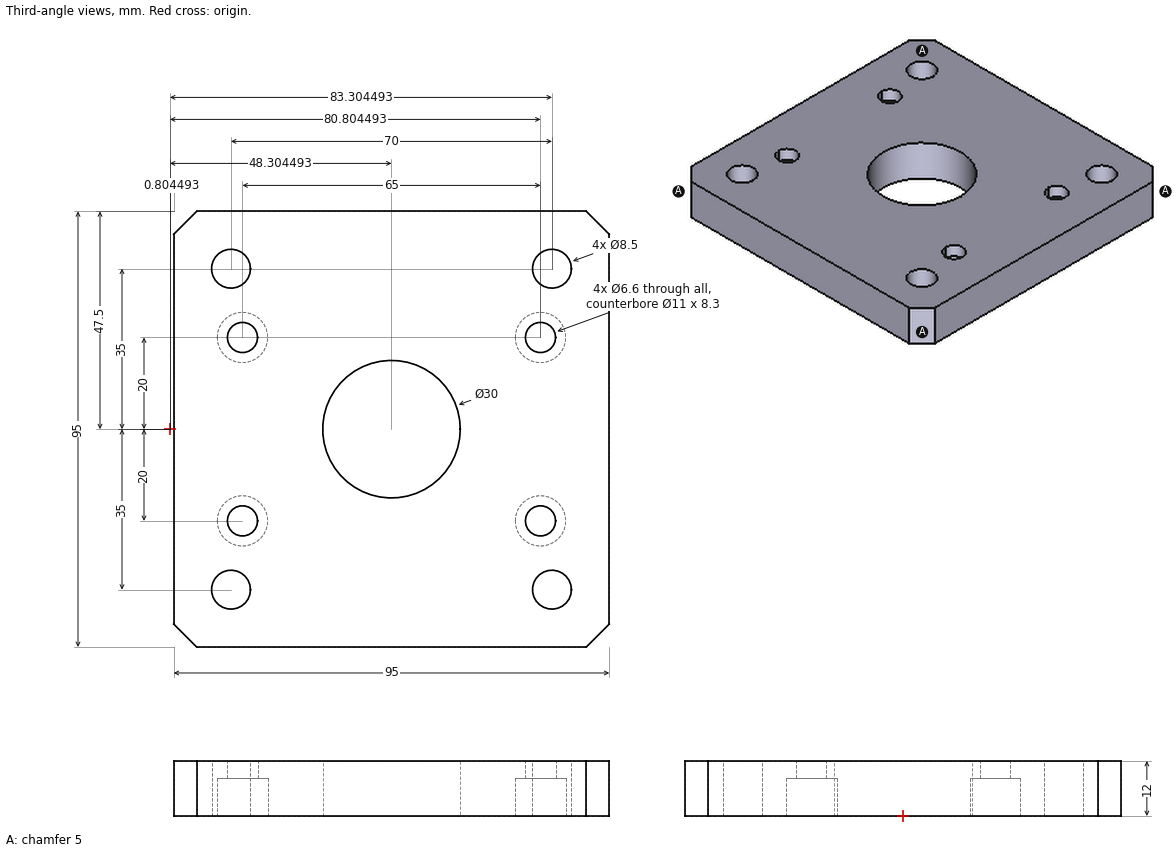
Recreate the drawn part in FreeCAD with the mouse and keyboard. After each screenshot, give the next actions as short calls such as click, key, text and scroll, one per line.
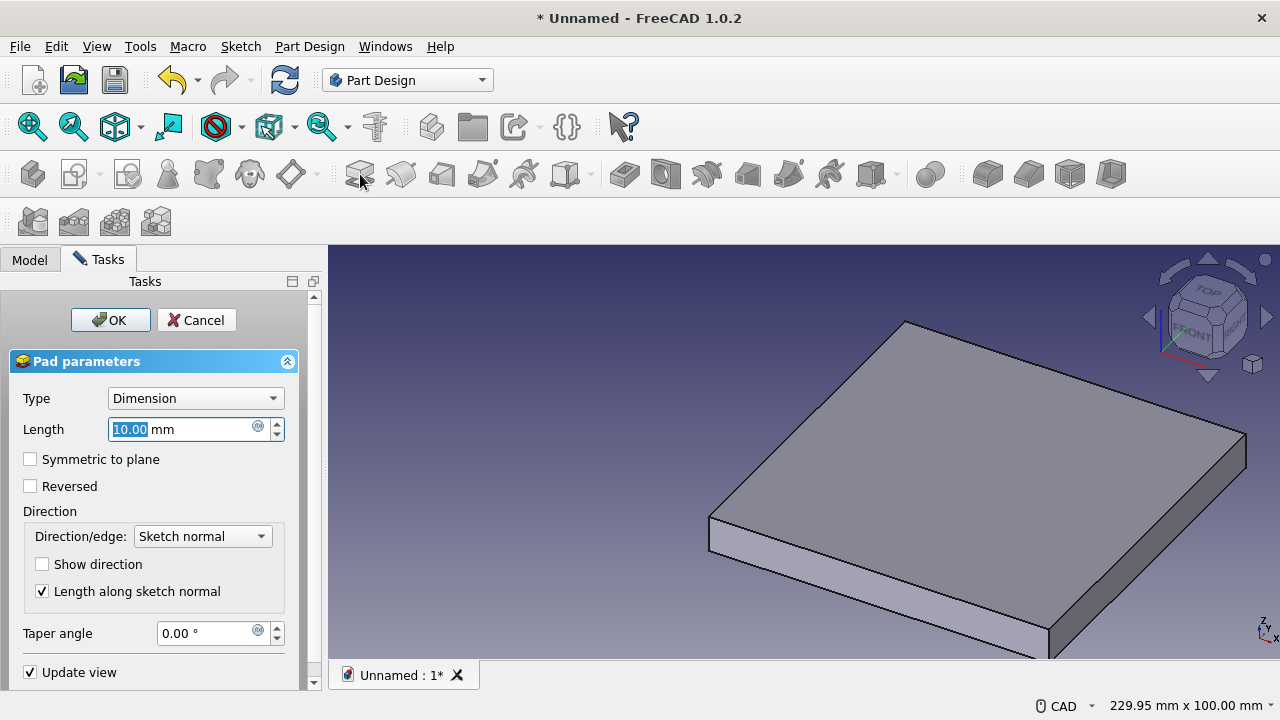
text(12)
key(Tab)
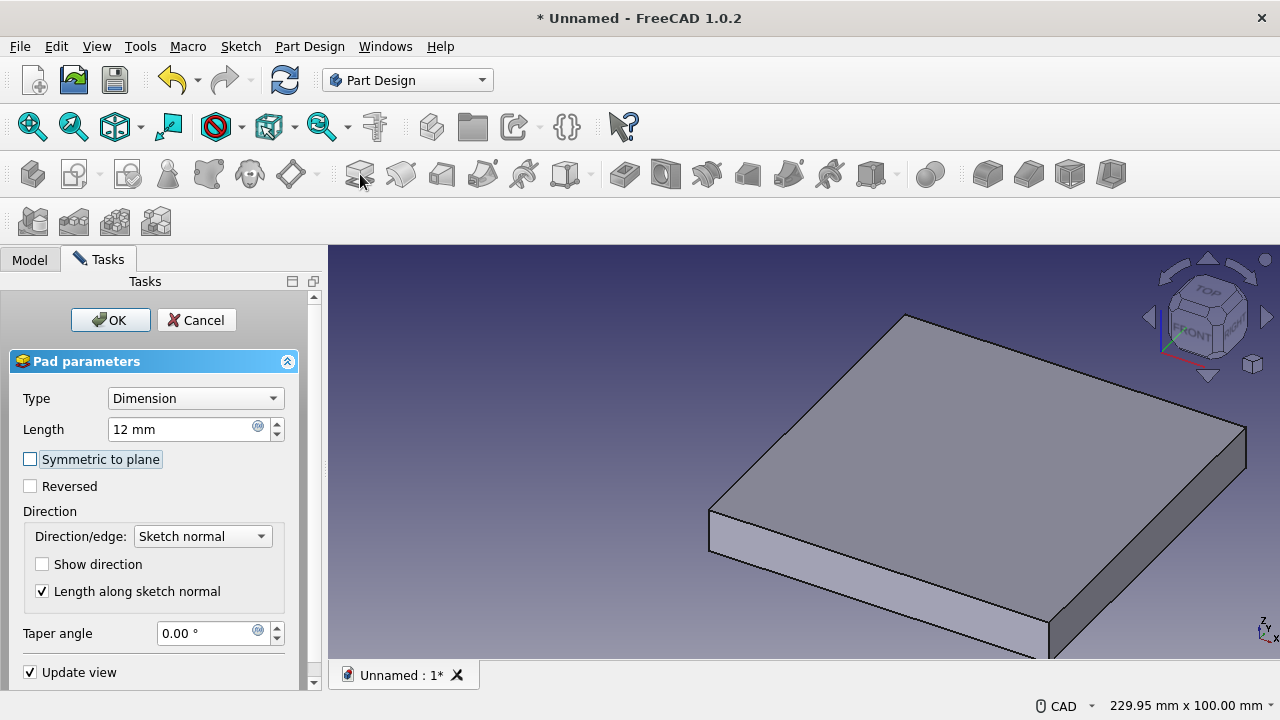
click(111, 320)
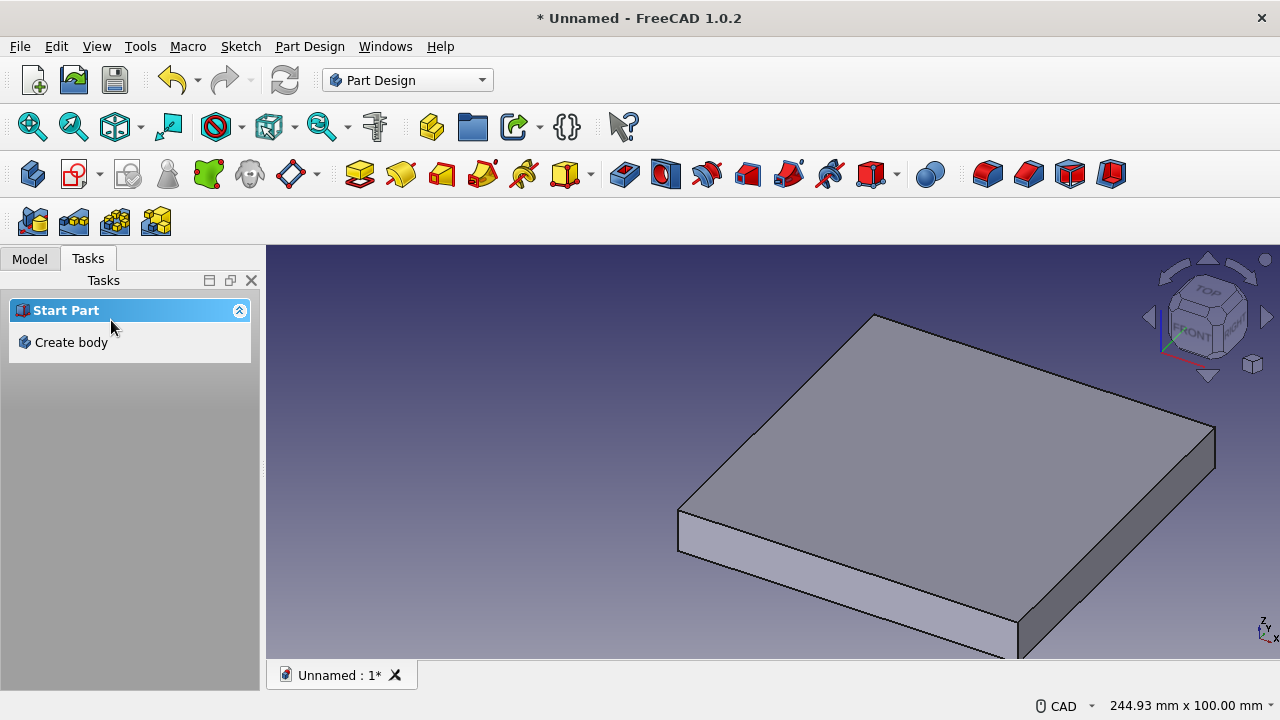
key(v)
key(f)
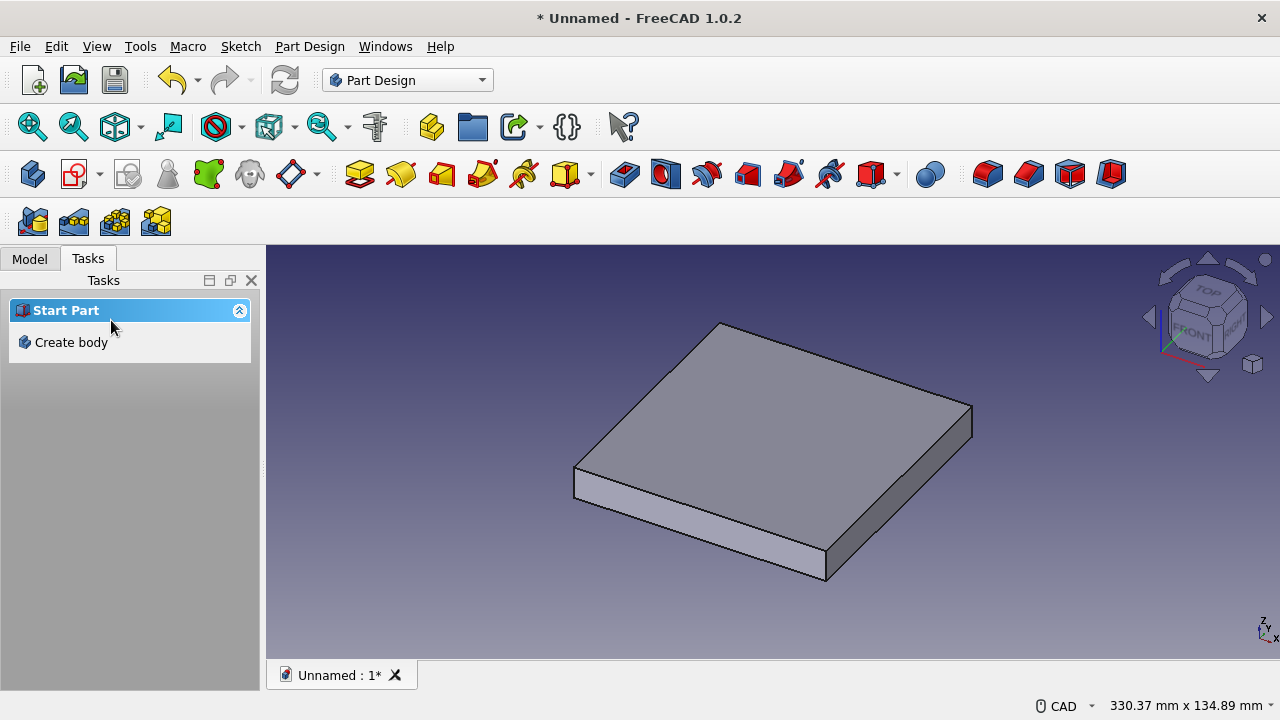
click(773, 436)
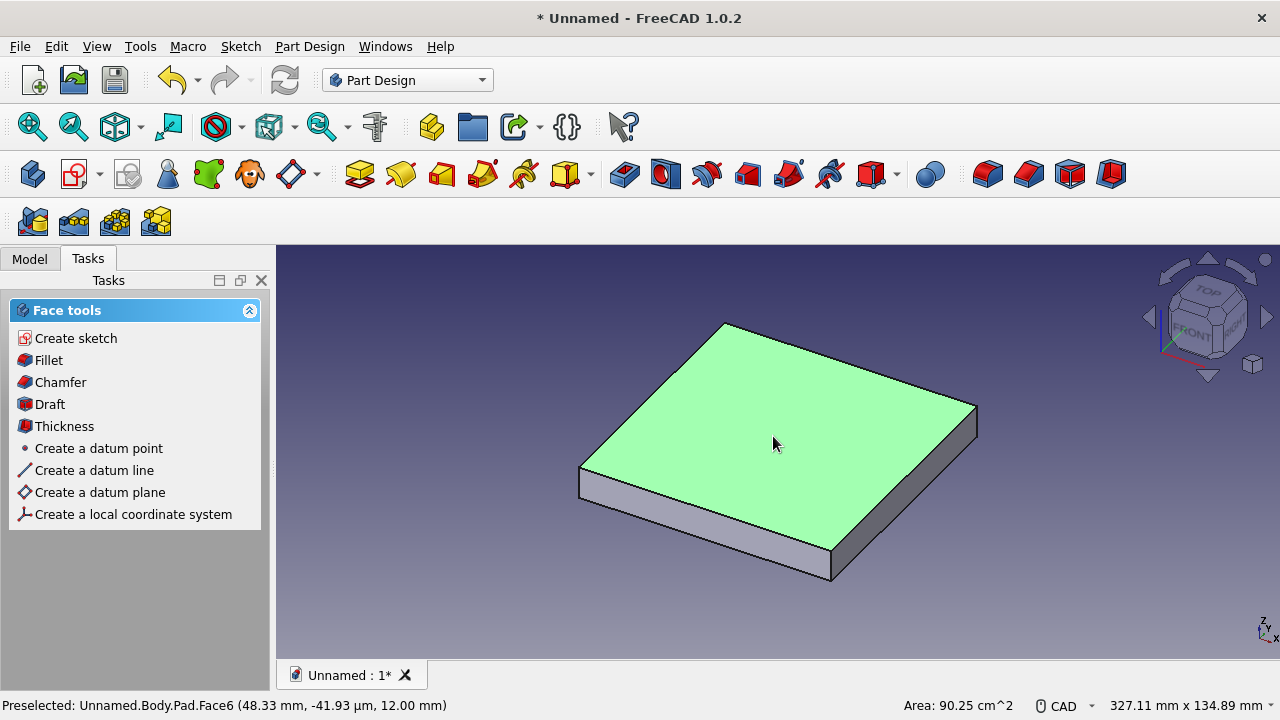
click(74, 174)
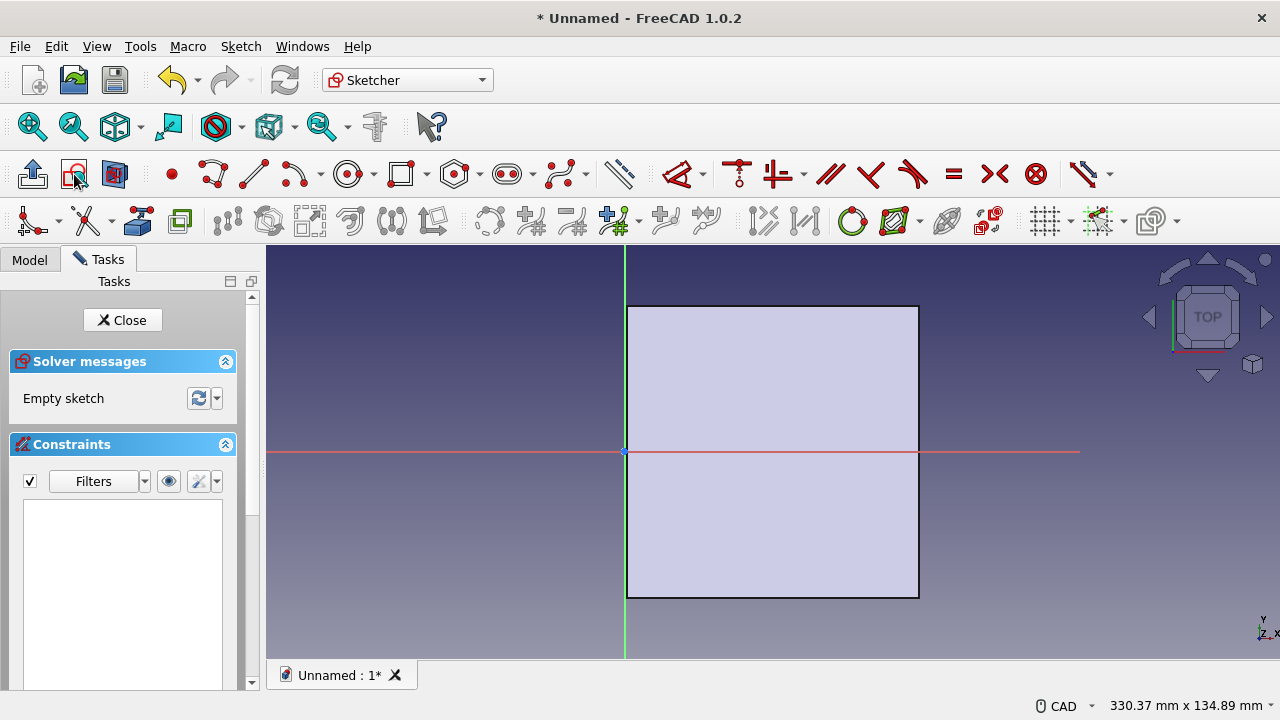
scroll(732, 452, up, 5)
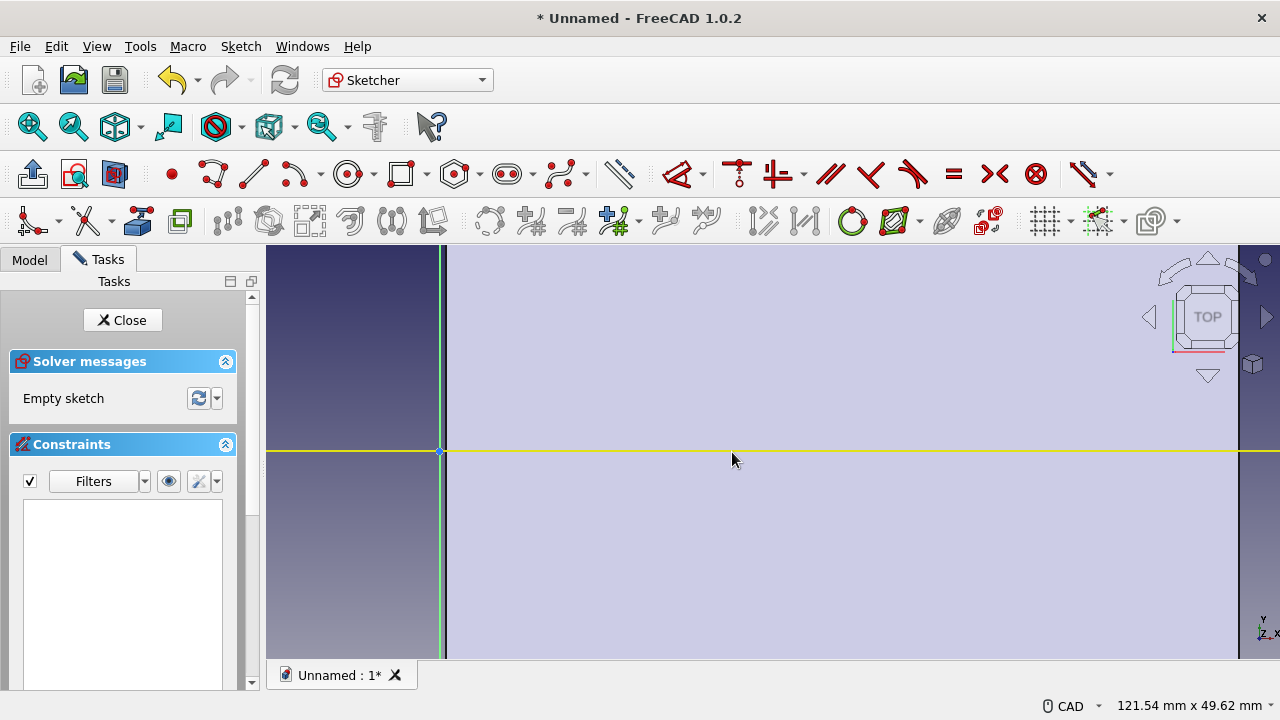
click(348, 174)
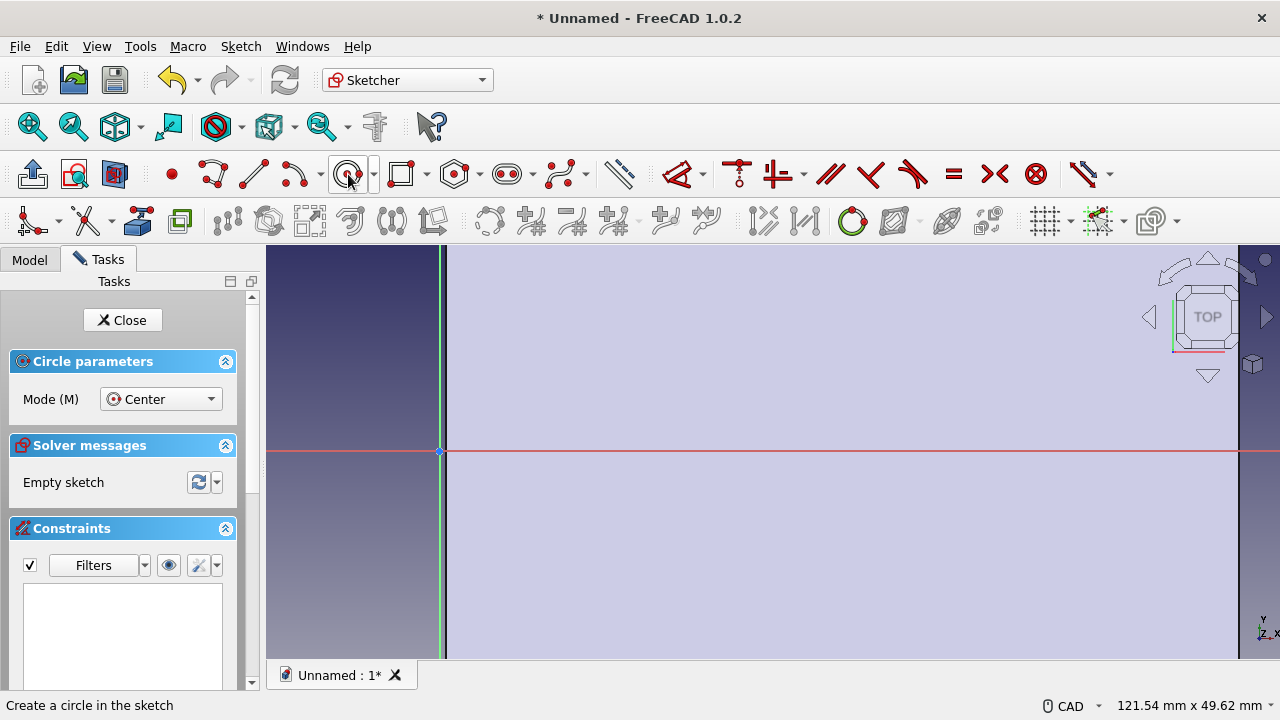
click(843, 451)
click(931, 363)
key(Escape)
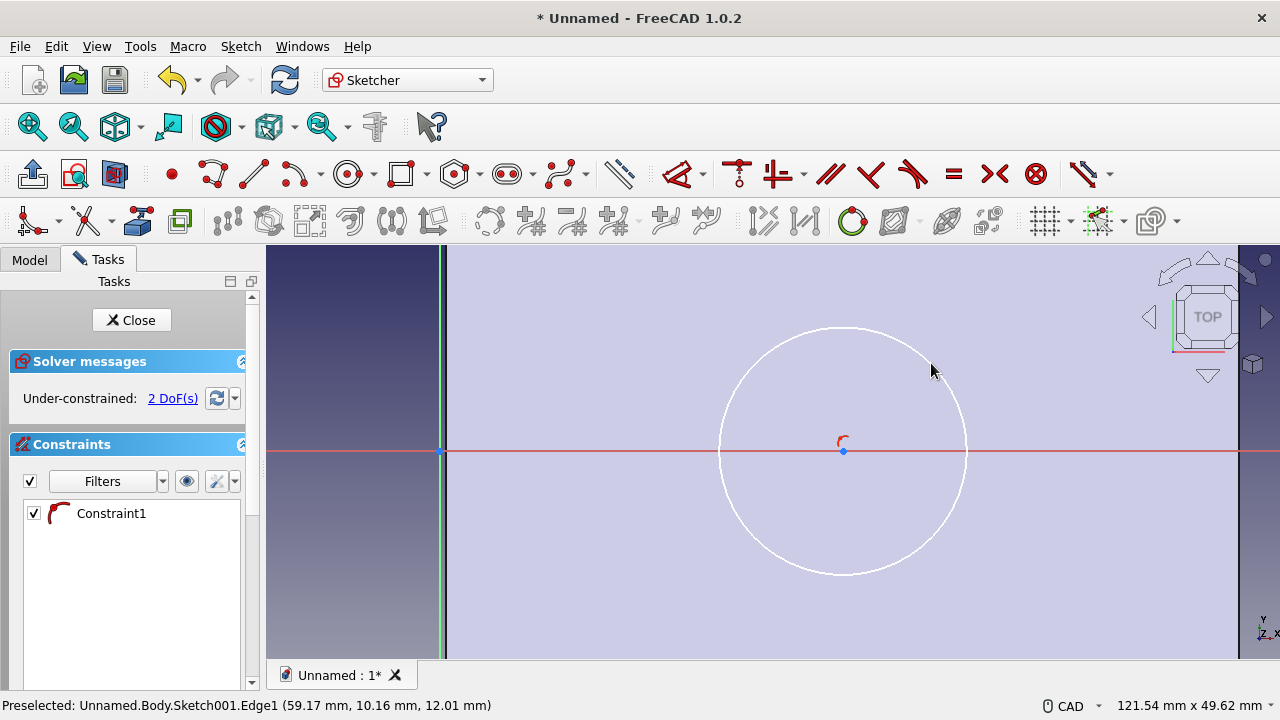
key(d)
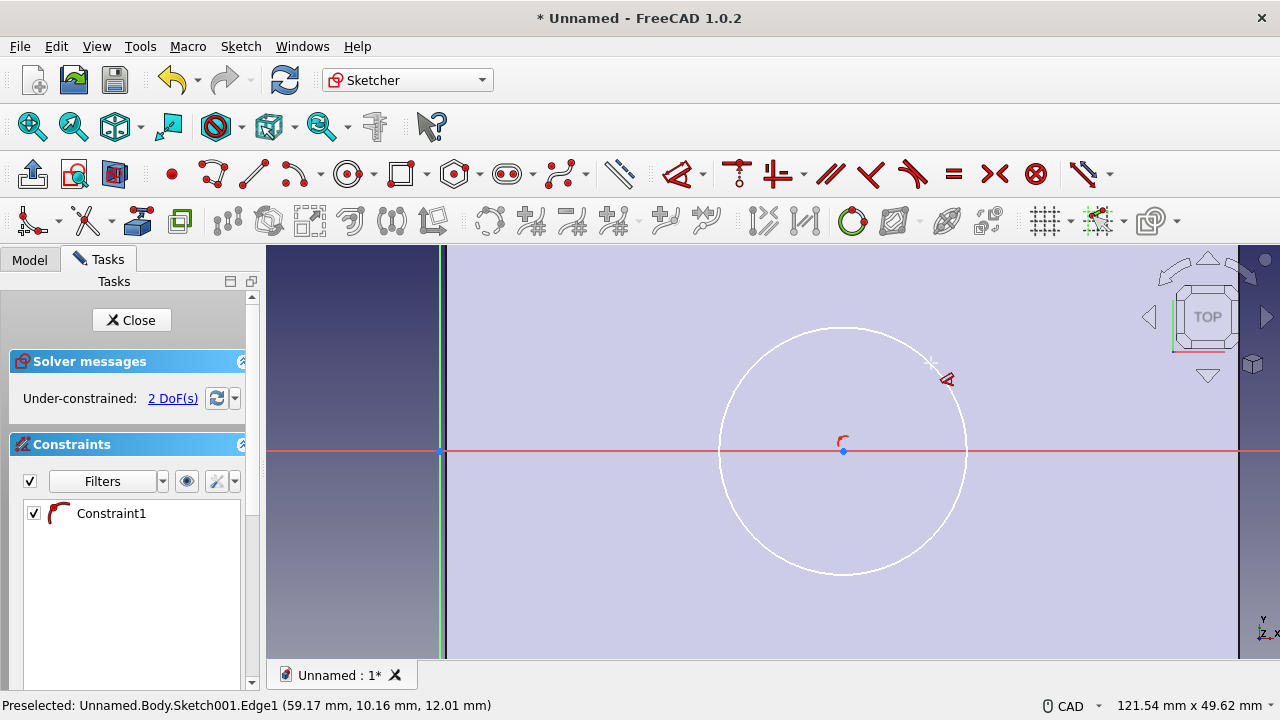
click(930, 363)
click(952, 340)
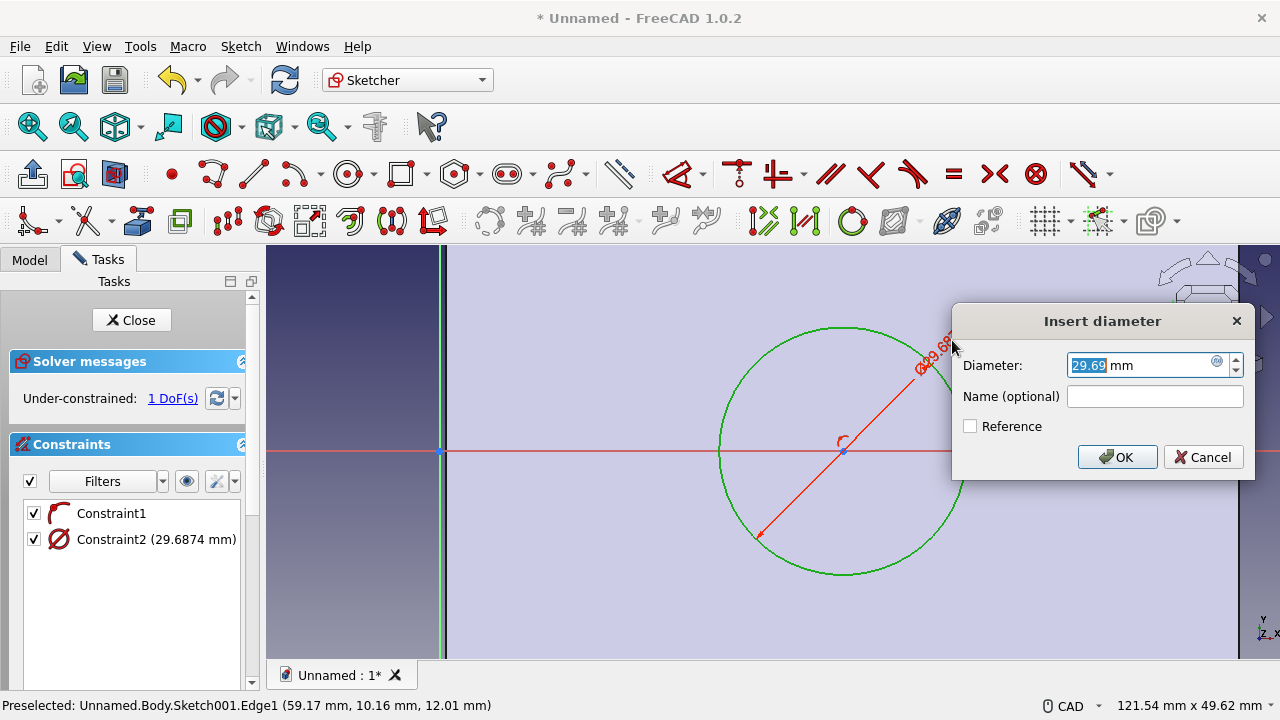
text(30)
key(Return)